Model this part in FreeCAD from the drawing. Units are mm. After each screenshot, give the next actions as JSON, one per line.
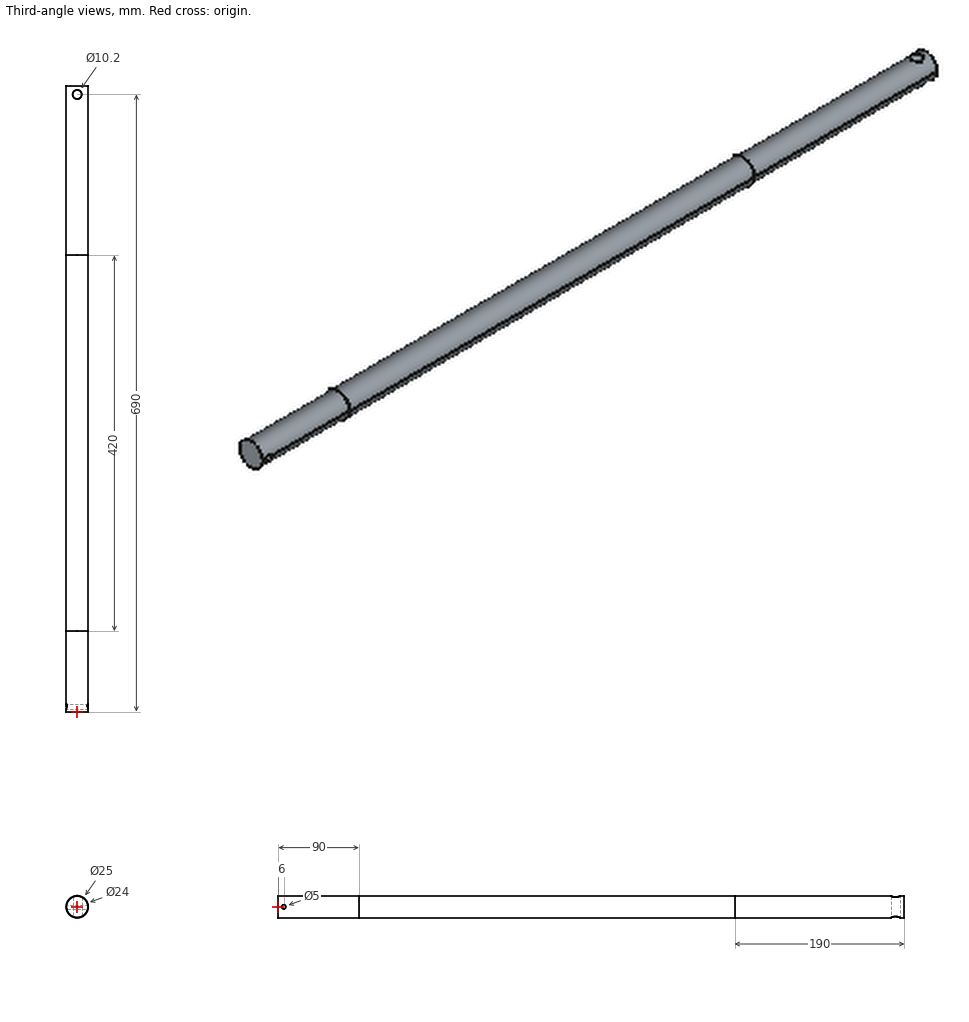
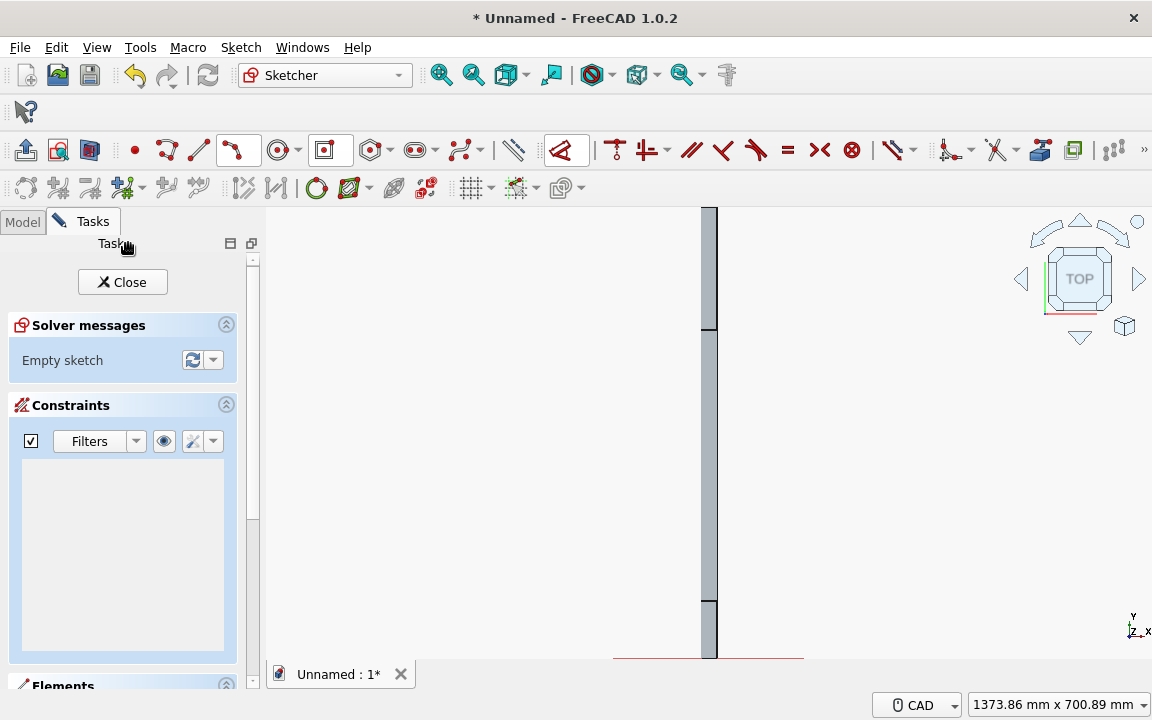
{"action": "left_click", "coordinate": [90, 150]}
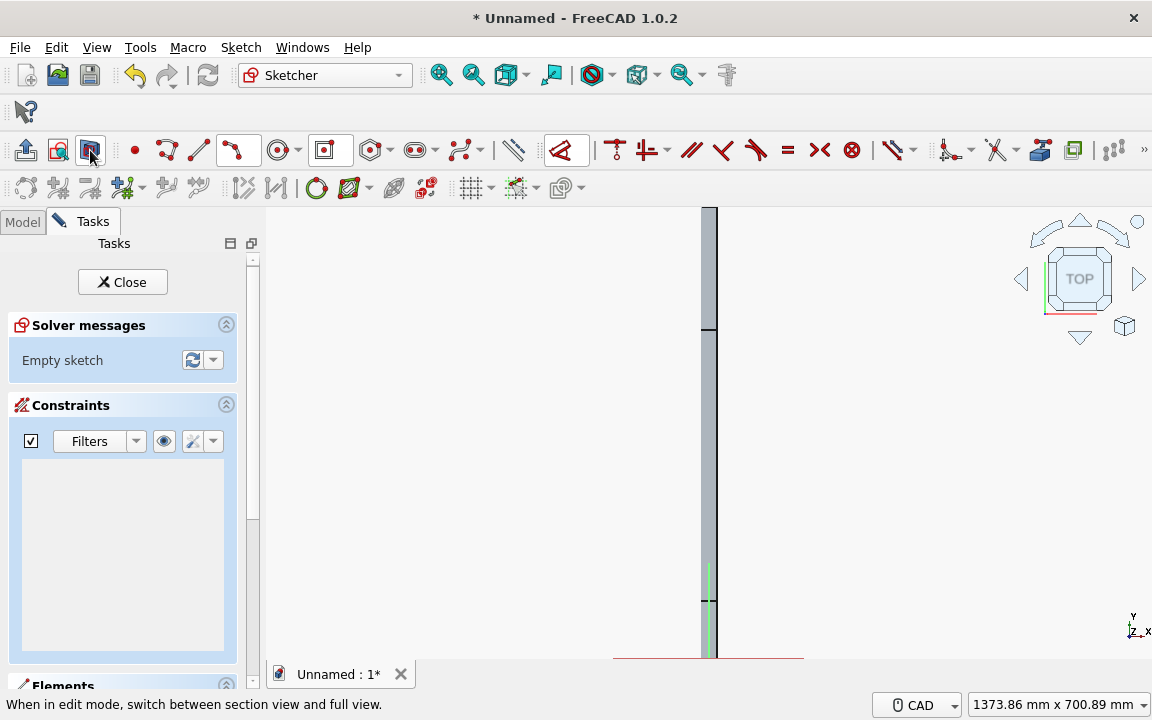
{"action": "scroll", "coordinate": [640, 433], "scroll_direction": "down", "scroll_amount": 5}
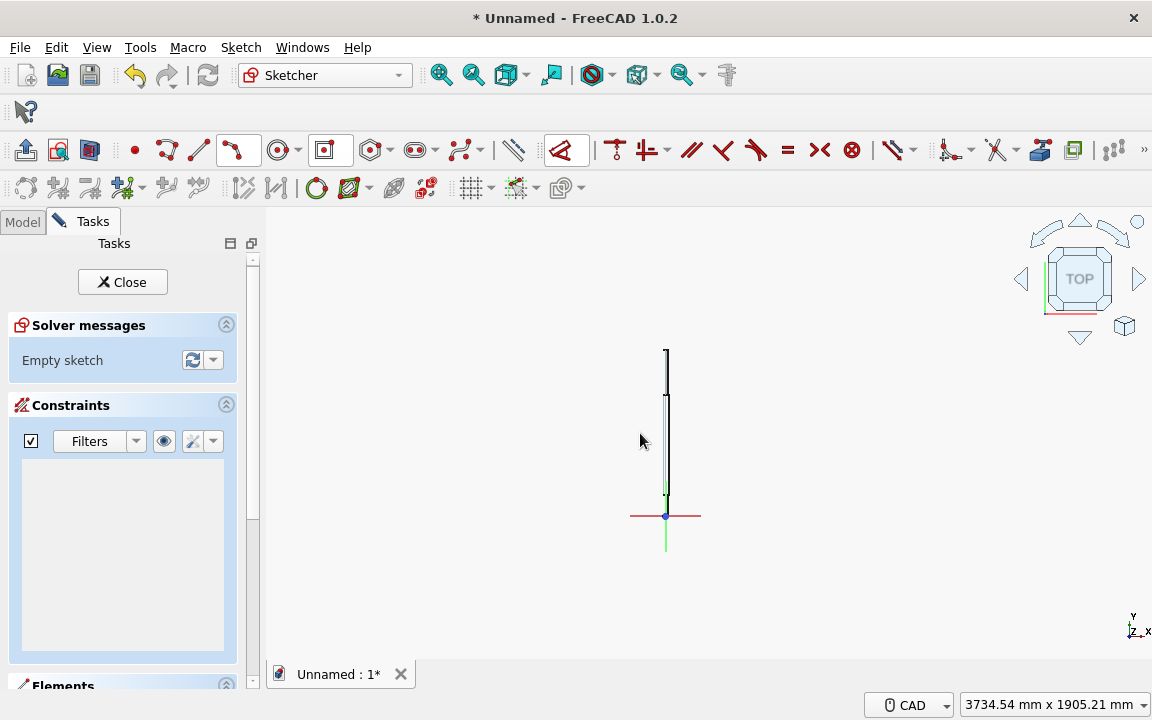
{"action": "scroll", "coordinate": [667, 348], "scroll_direction": "up", "scroll_amount": 15}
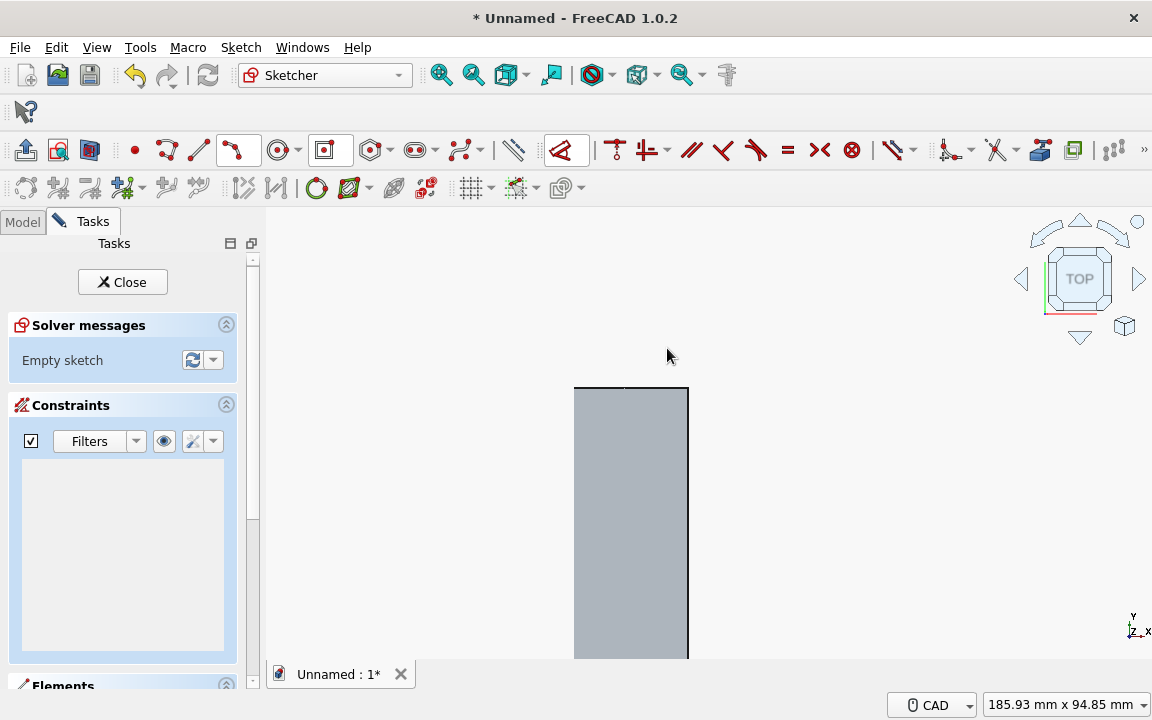
{"action": "scroll", "coordinate": [629, 436], "scroll_direction": "up", "scroll_amount": 9}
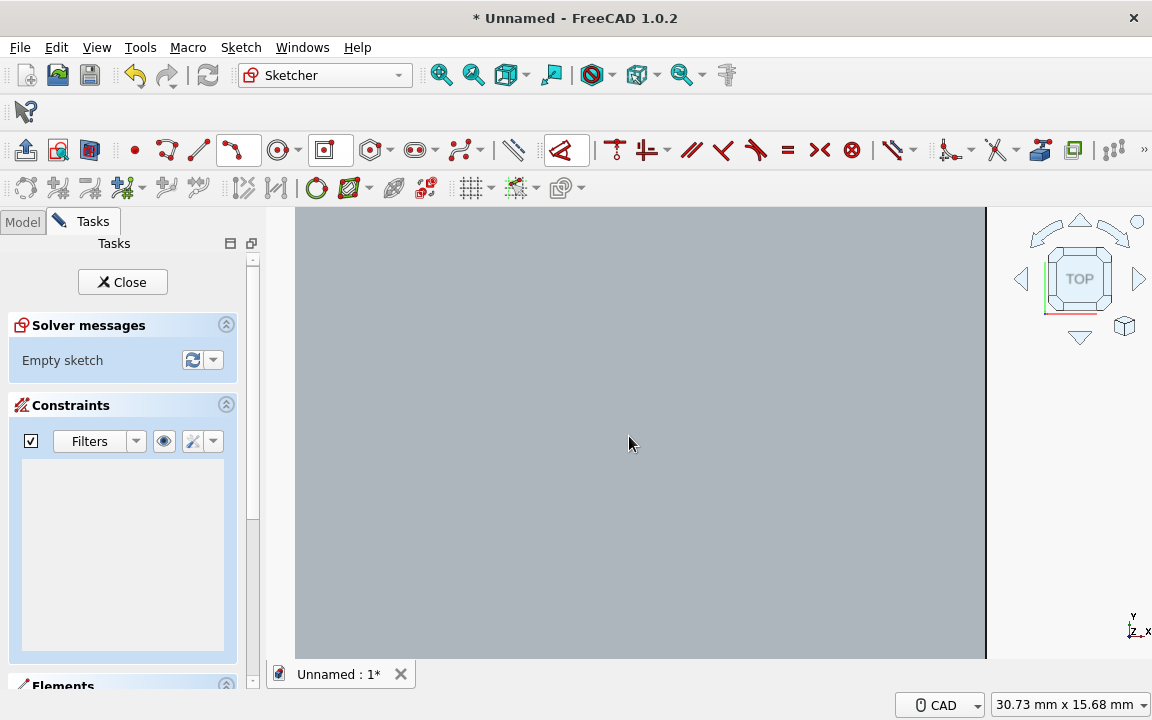
{"action": "key", "text": "g c"}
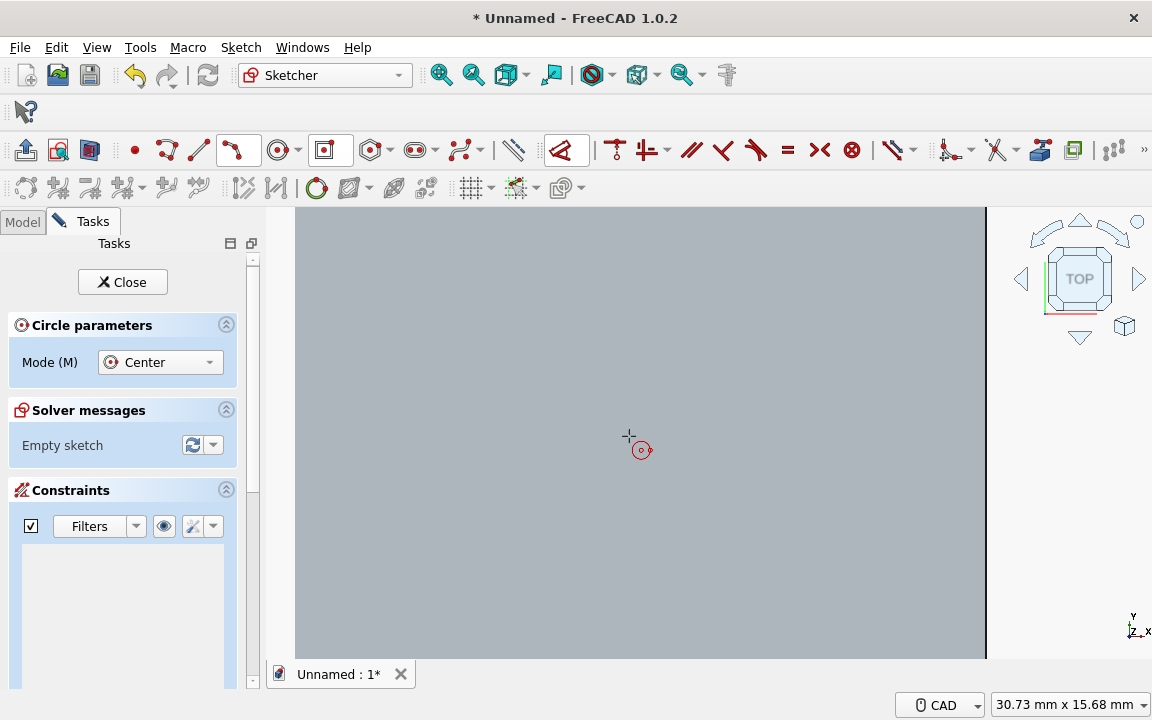
{"action": "left_click", "coordinate": [641, 430]}
{"action": "left_click", "coordinate": [745, 326]}
{"action": "key", "text": "Escape"}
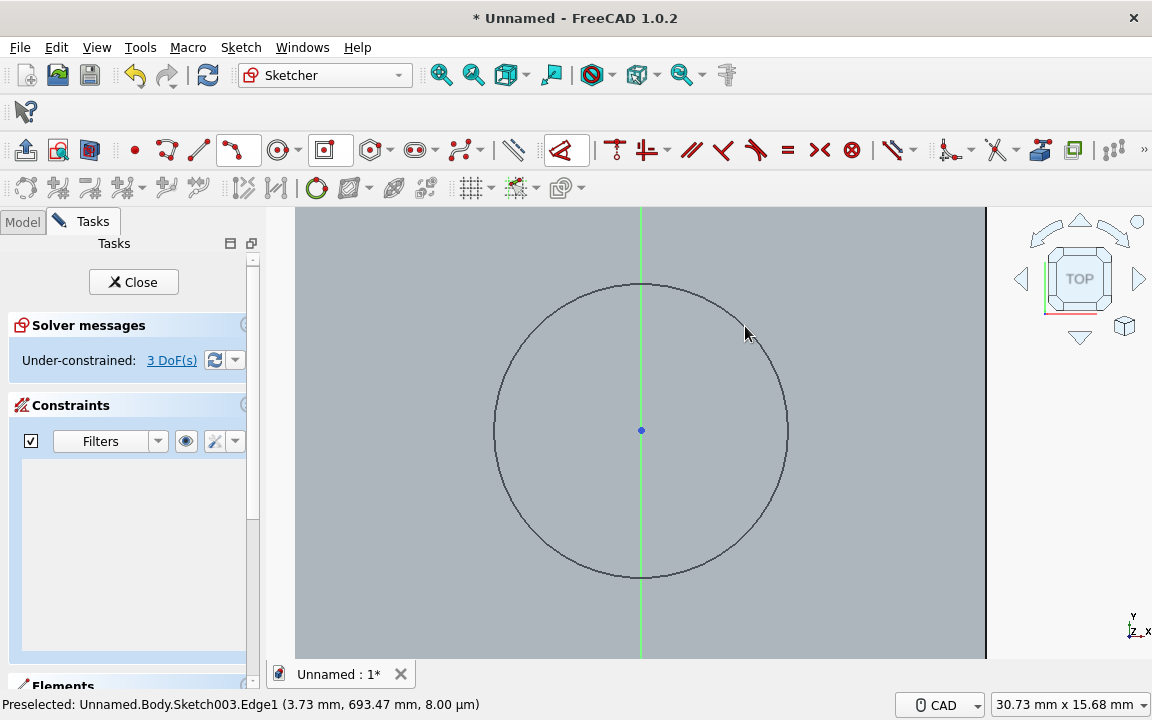
{"action": "left_click", "coordinate": [641, 431]}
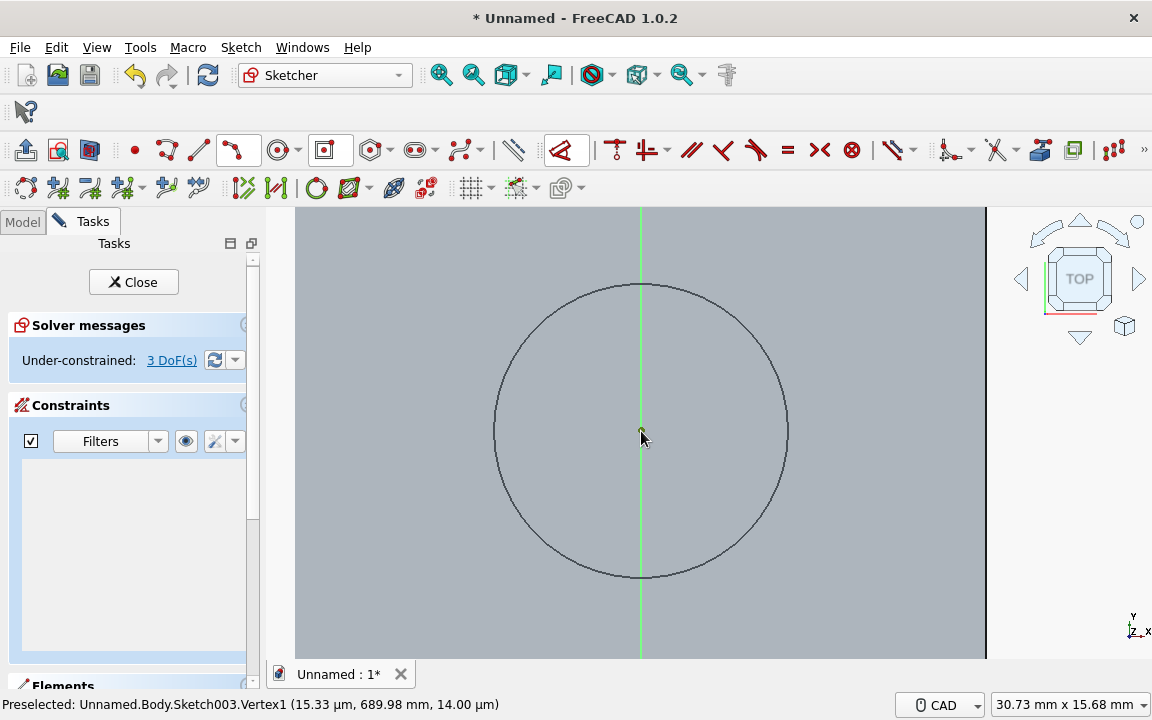
{"action": "left_click", "coordinate": [641, 546]}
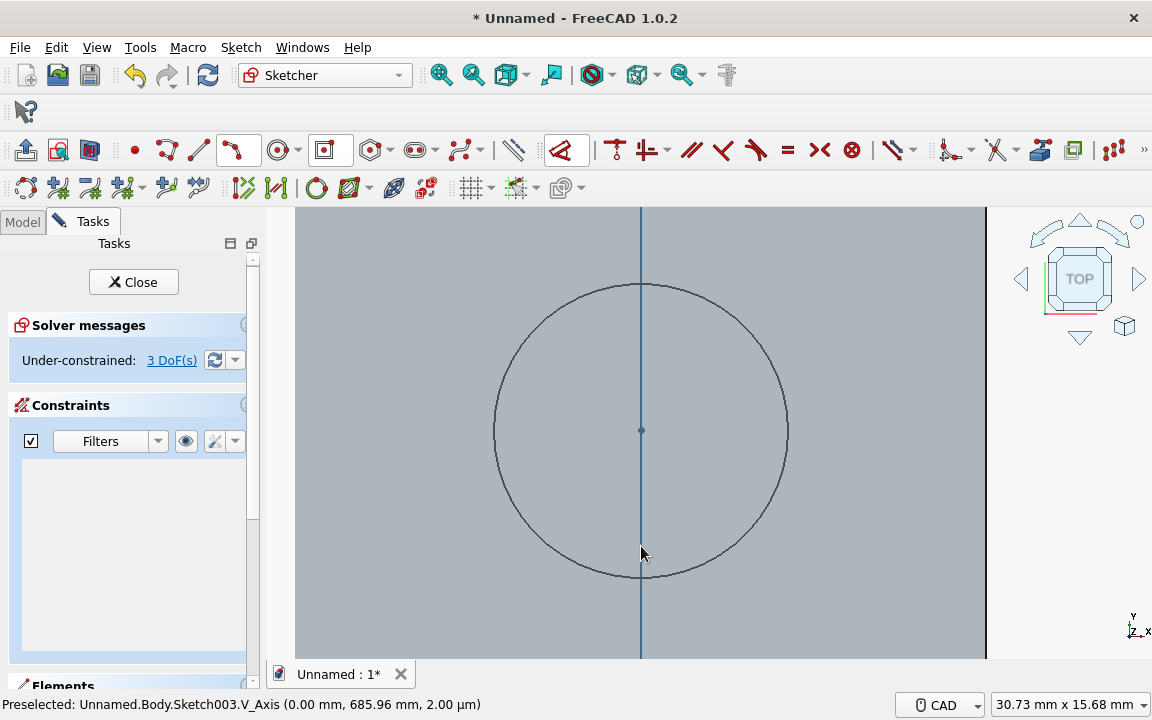
{"action": "key", "text": "c"}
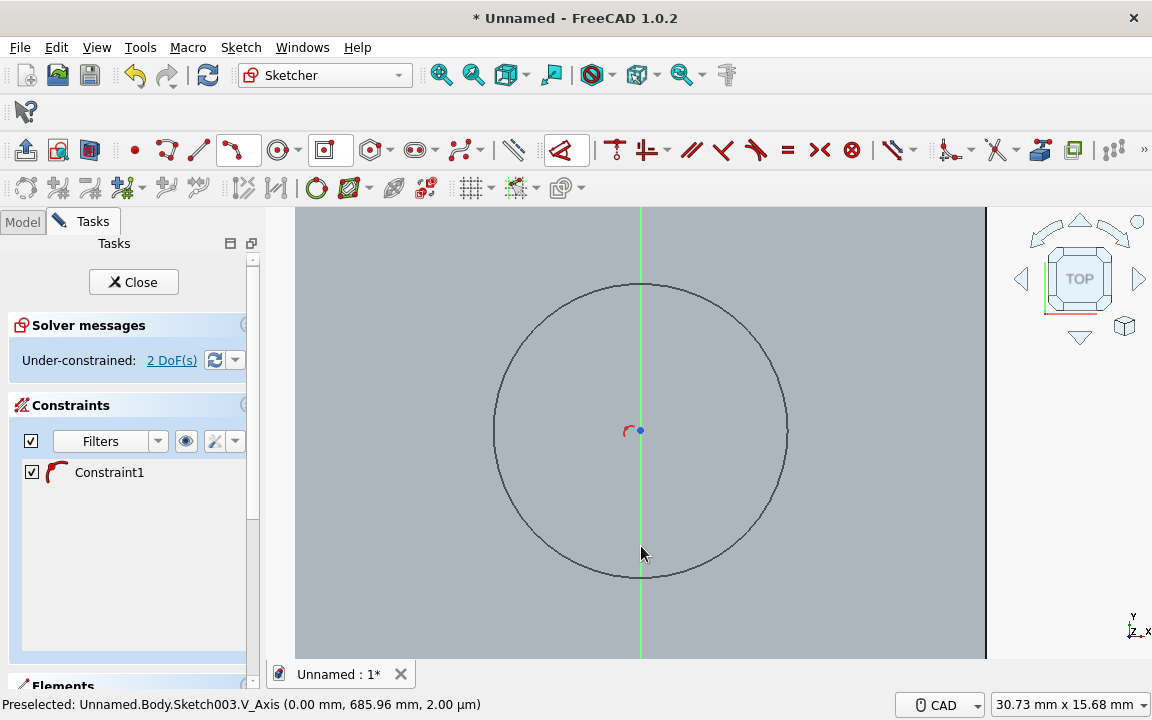
{"action": "left_click", "coordinate": [744, 327]}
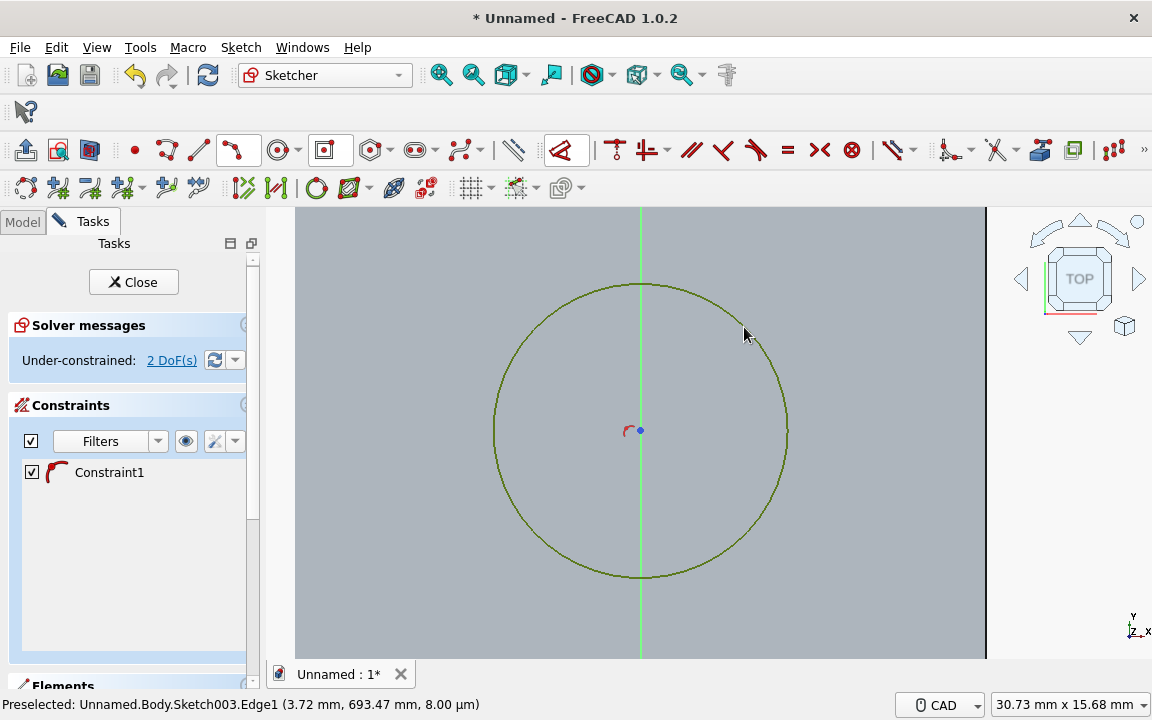
{"action": "left_click", "coordinate": [584, 150]}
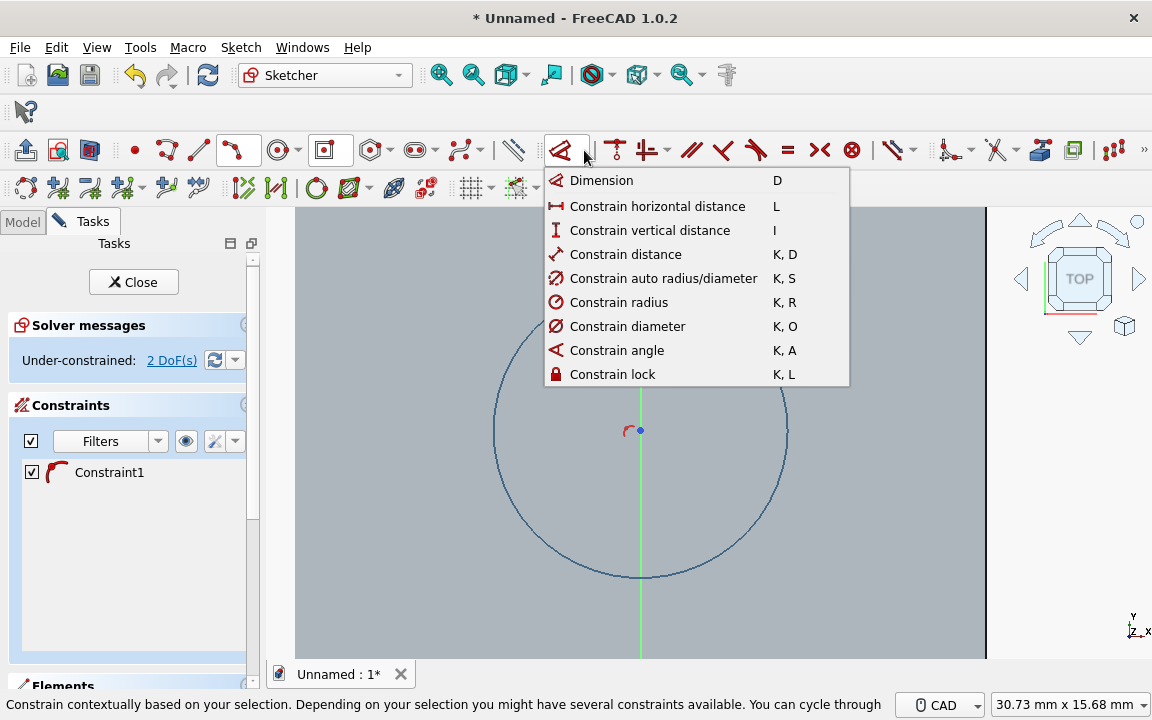
{"action": "left_click", "coordinate": [697, 326]}